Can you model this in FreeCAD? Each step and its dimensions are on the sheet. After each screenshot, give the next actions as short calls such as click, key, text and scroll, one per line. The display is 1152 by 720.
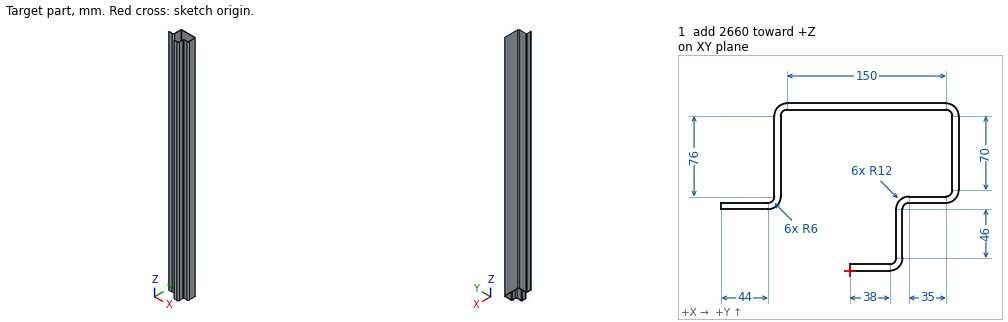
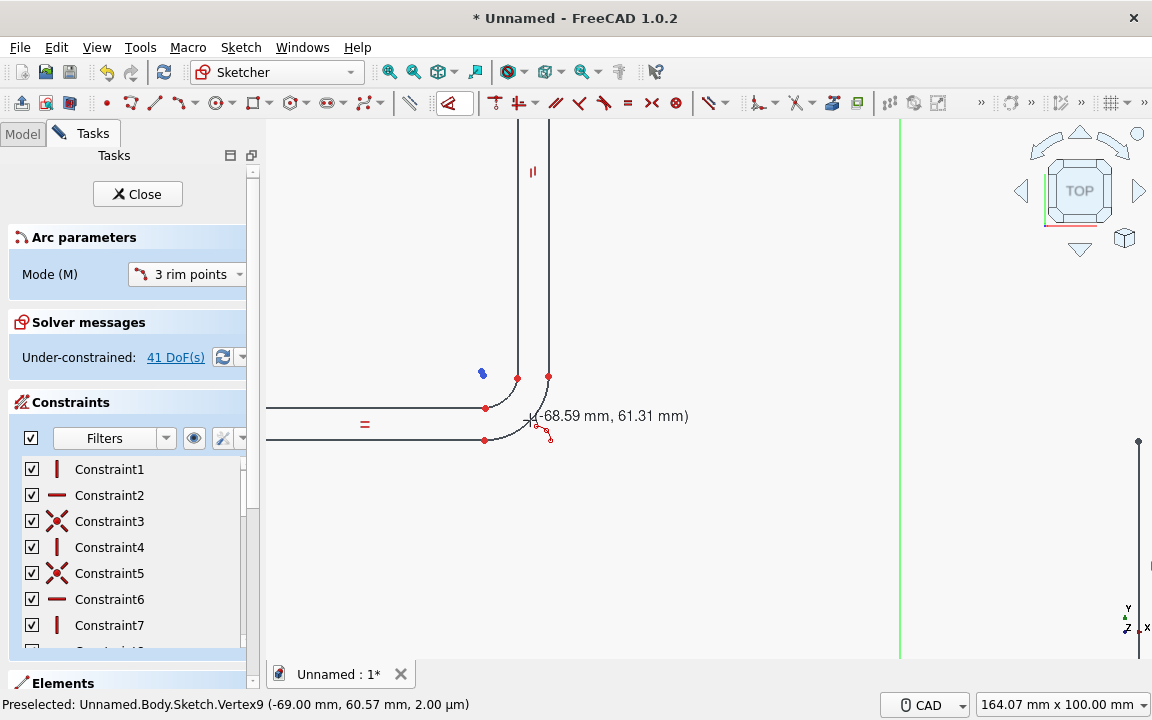
scroll(518, 426, down, 5)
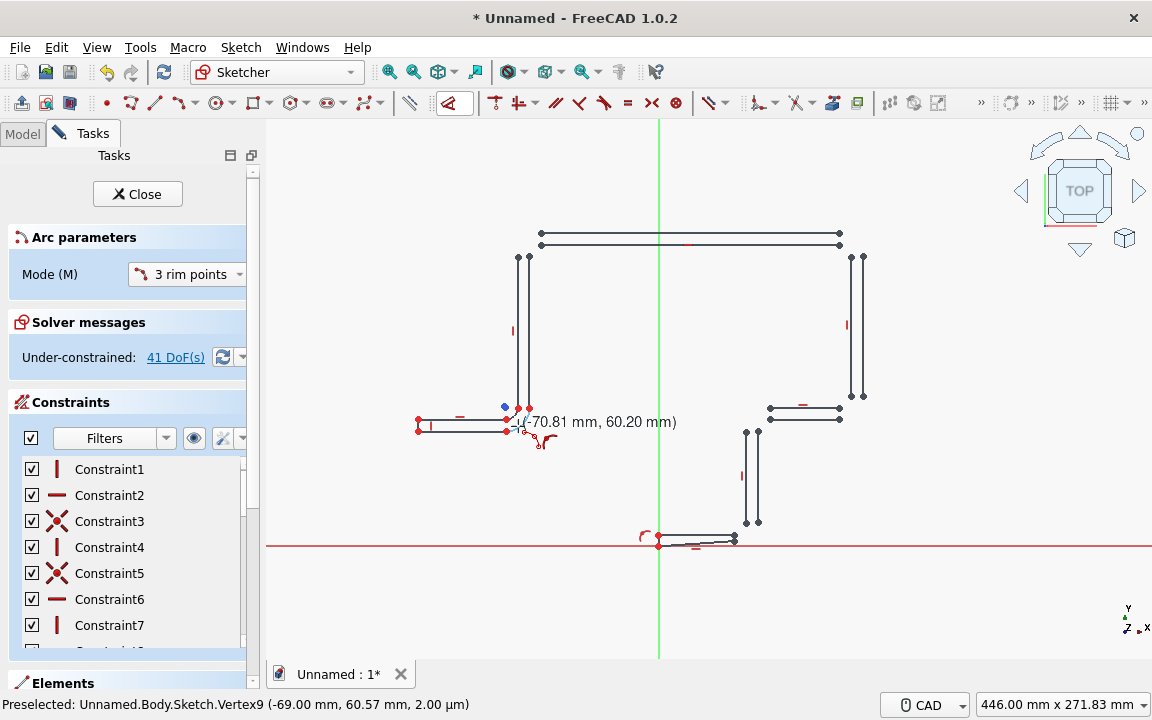
scroll(530, 256, up, 2)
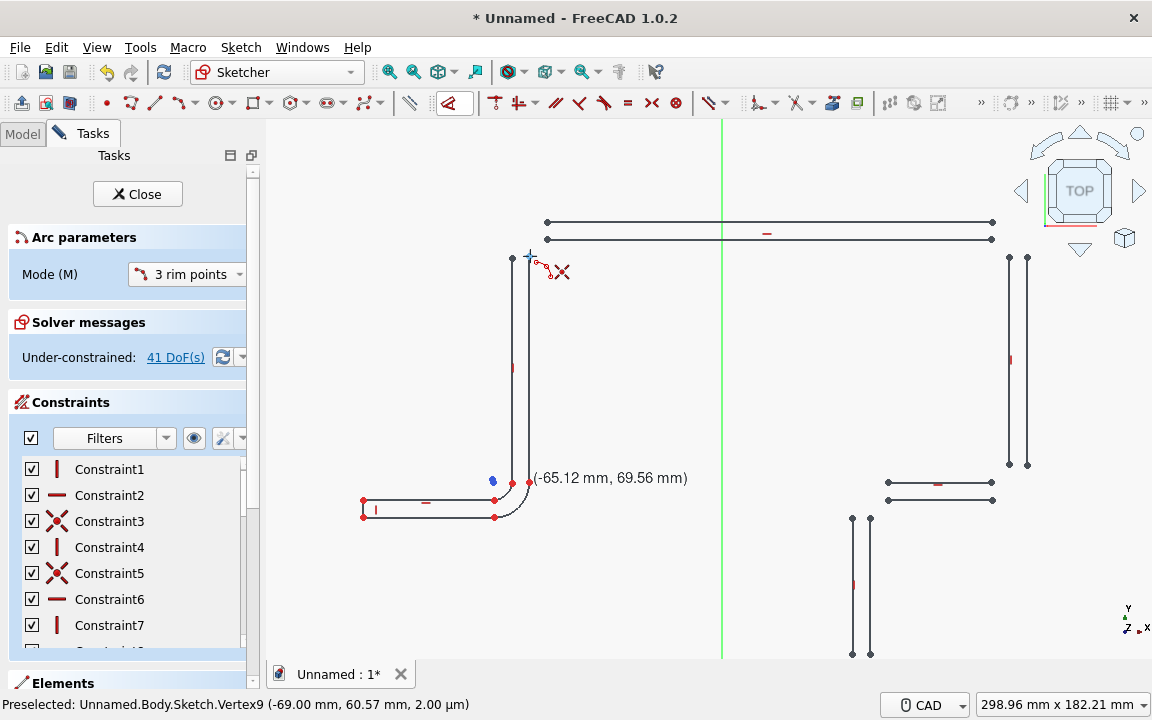
click(529, 257)
click(547, 240)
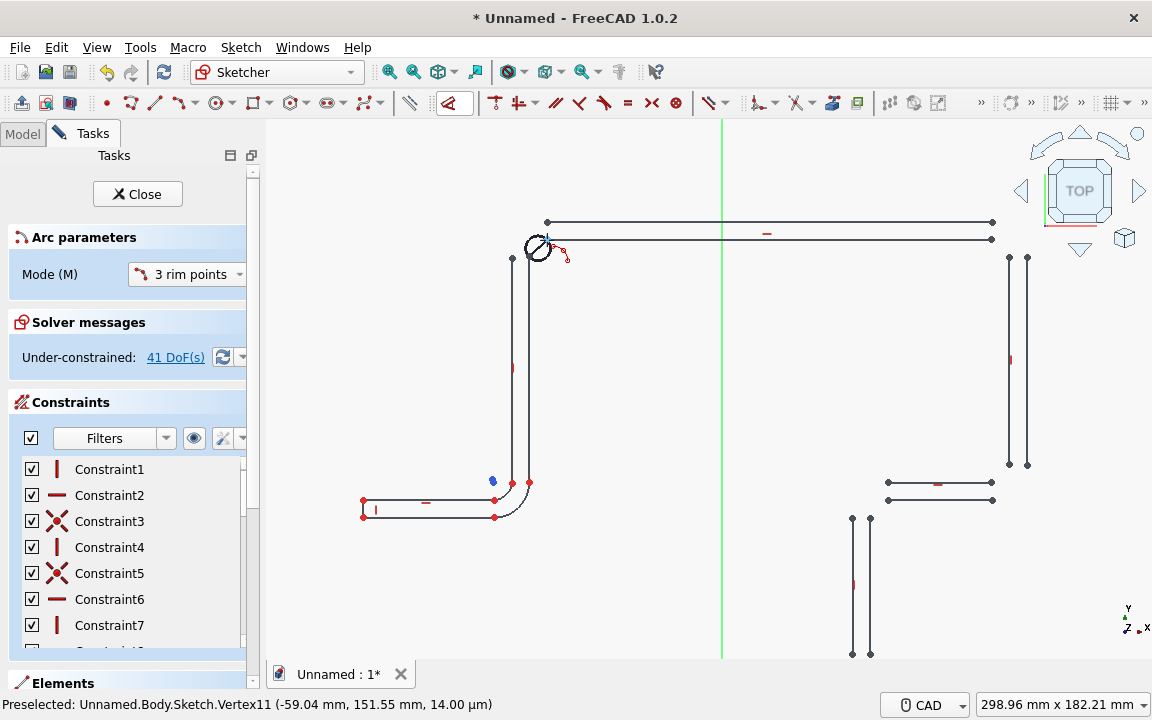
scroll(535, 244, up, 6)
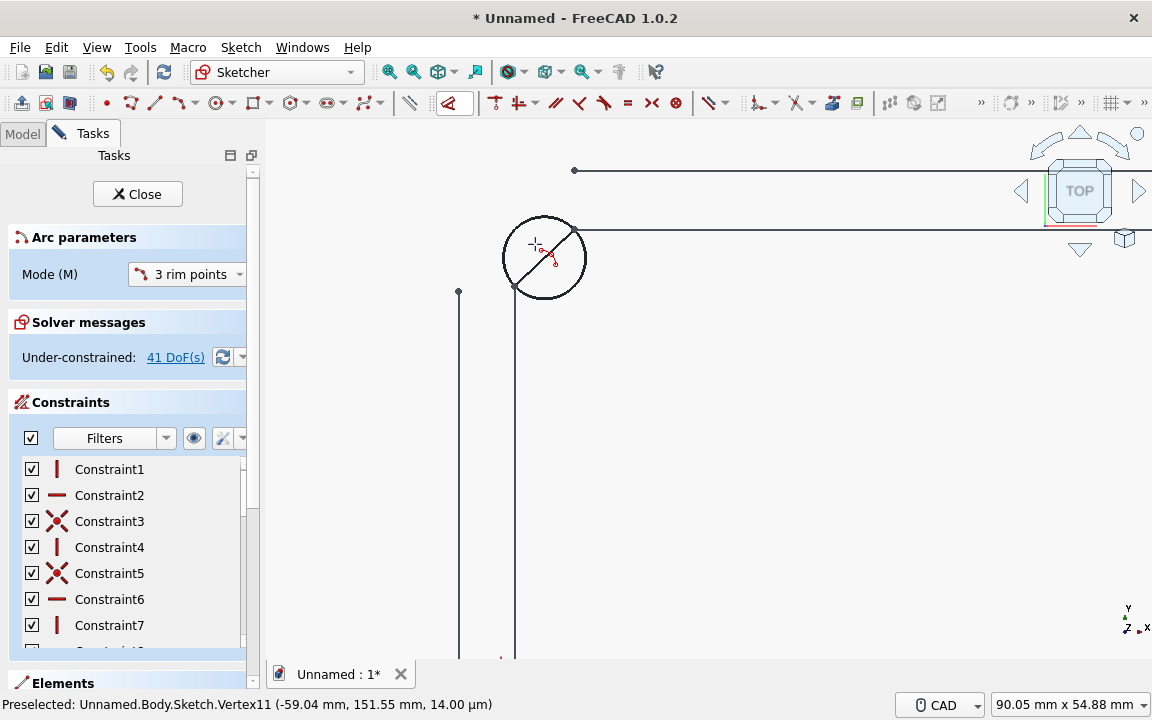
click(533, 243)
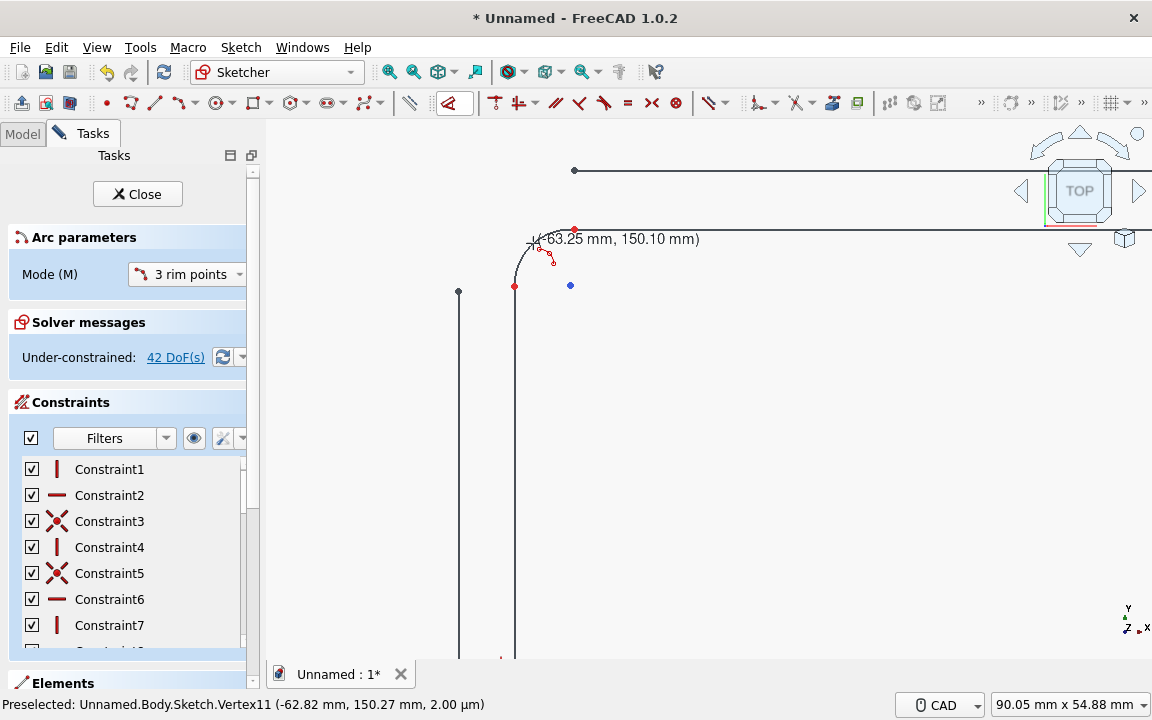
scroll(533, 249, down, 8)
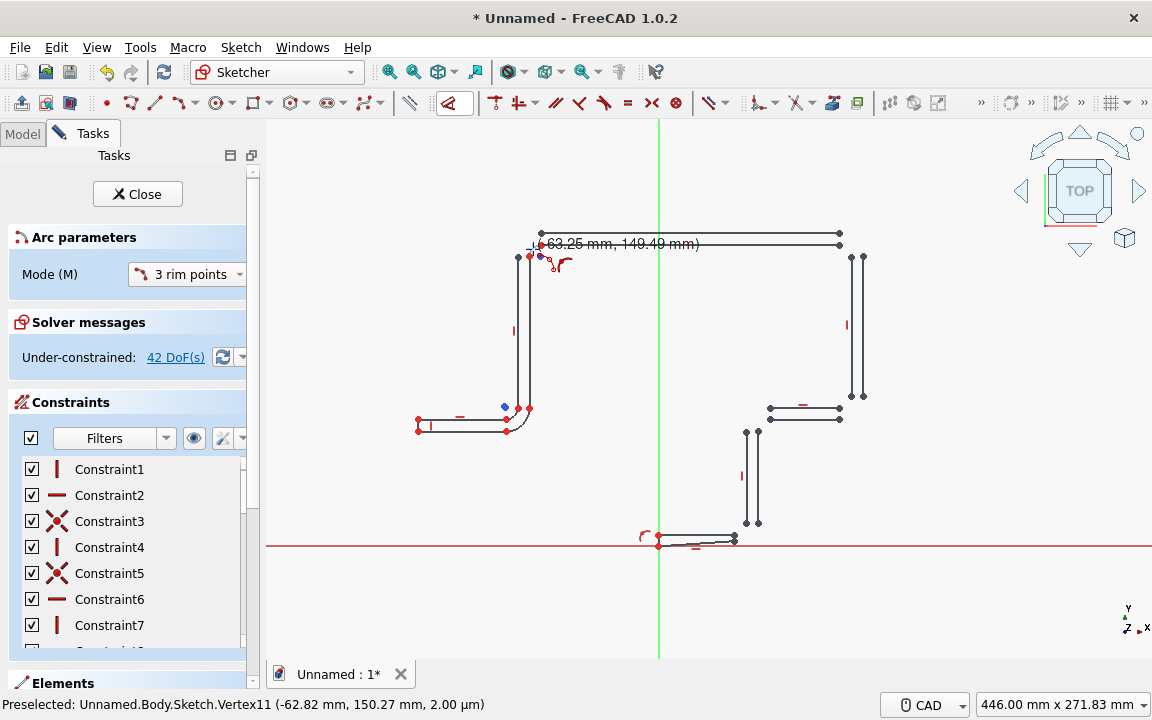
scroll(840, 244, up, 2)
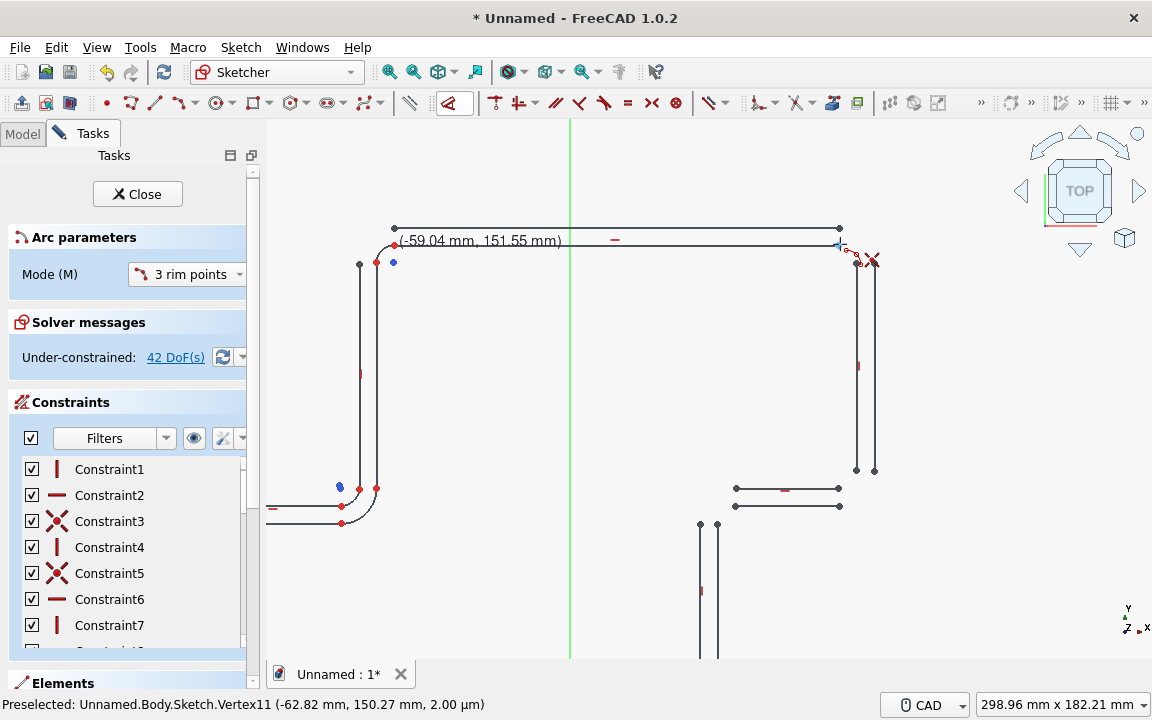
click(839, 246)
click(857, 264)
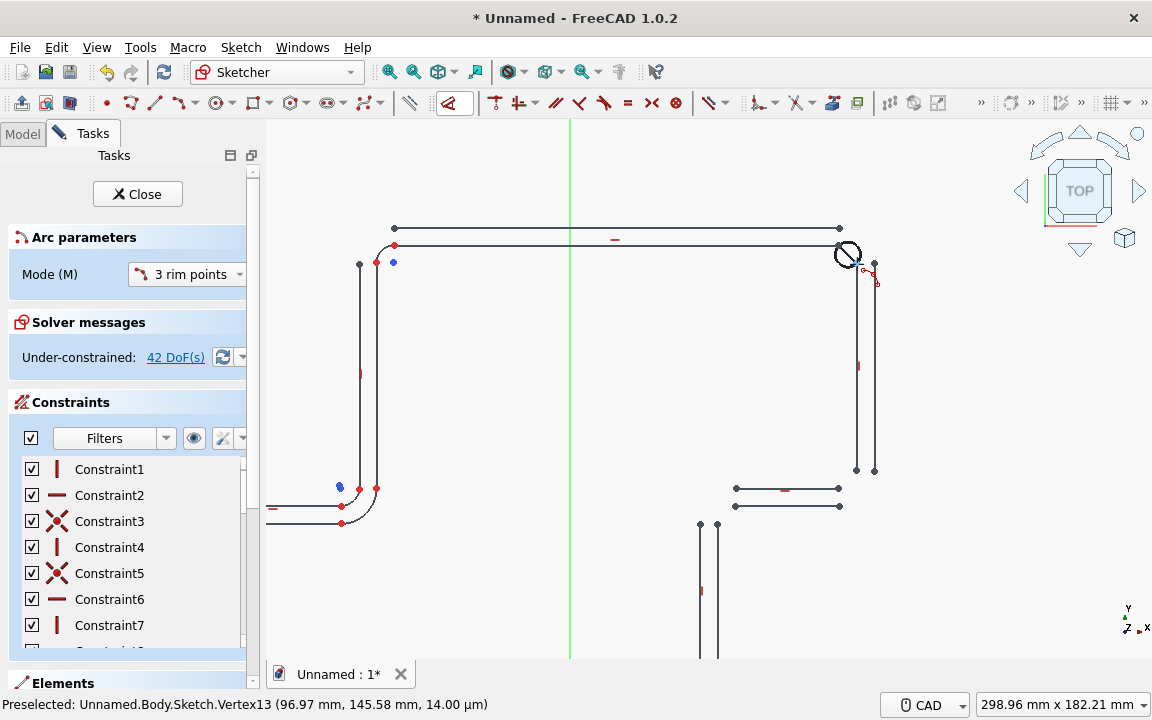
scroll(852, 250, up, 6)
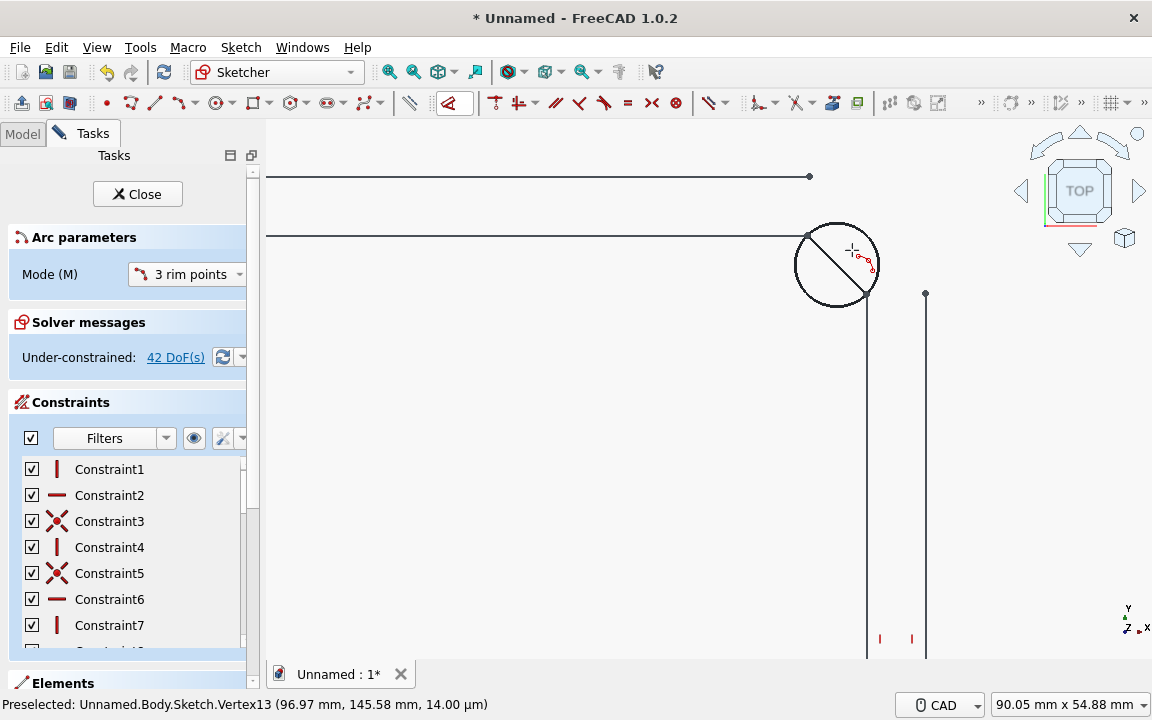
click(850, 248)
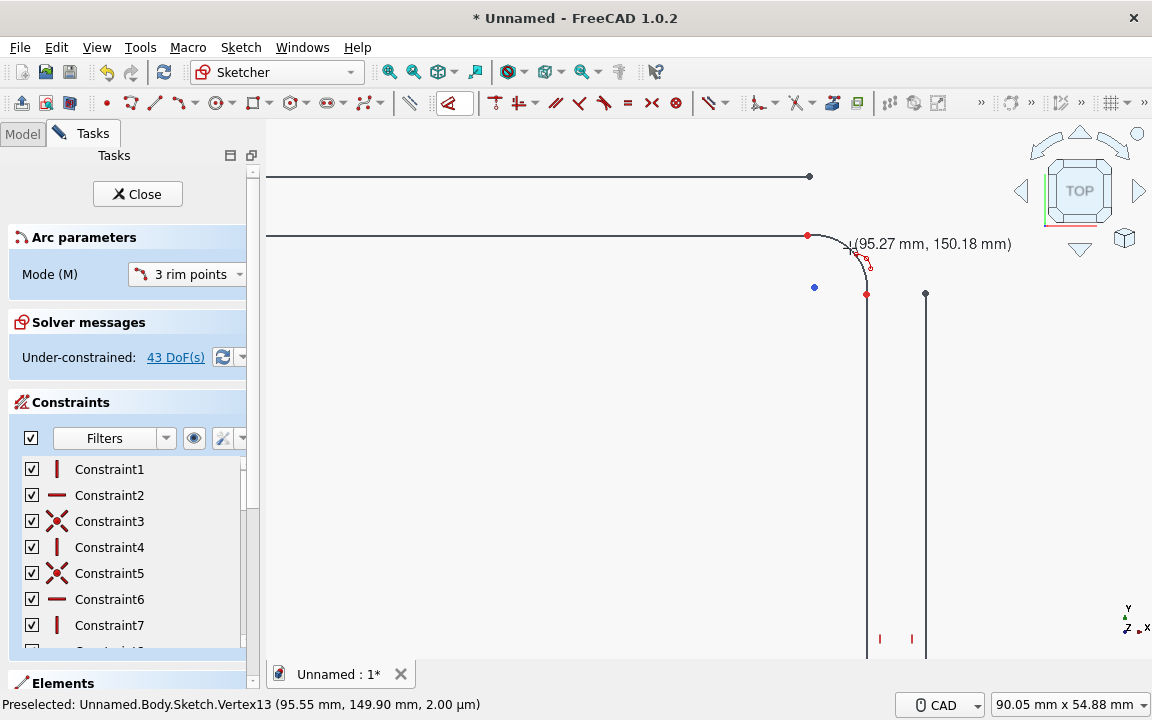
scroll(847, 247, down, 8)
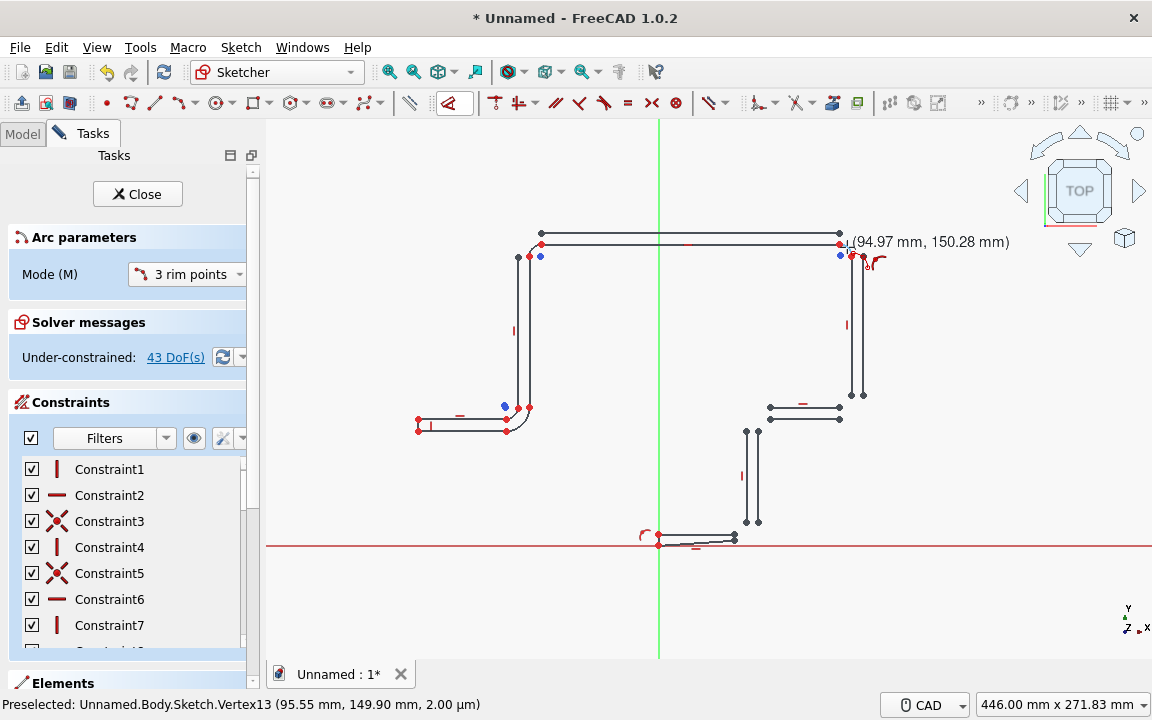
scroll(852, 395, up, 2)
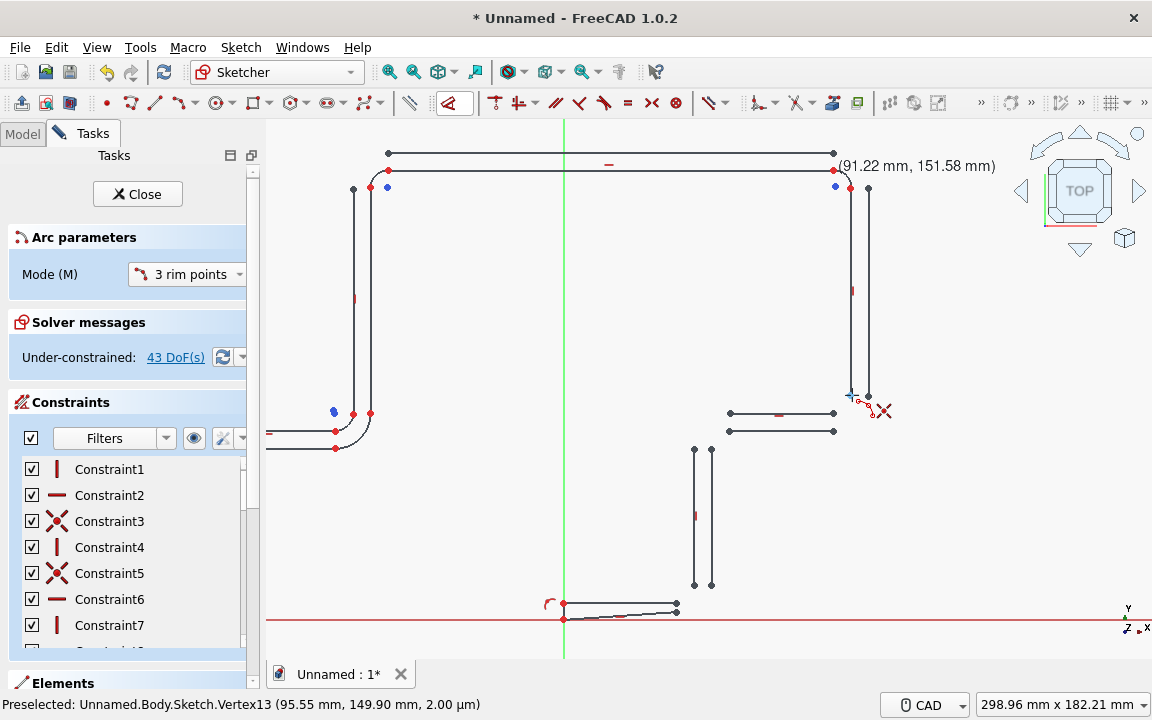
click(851, 396)
click(833, 414)